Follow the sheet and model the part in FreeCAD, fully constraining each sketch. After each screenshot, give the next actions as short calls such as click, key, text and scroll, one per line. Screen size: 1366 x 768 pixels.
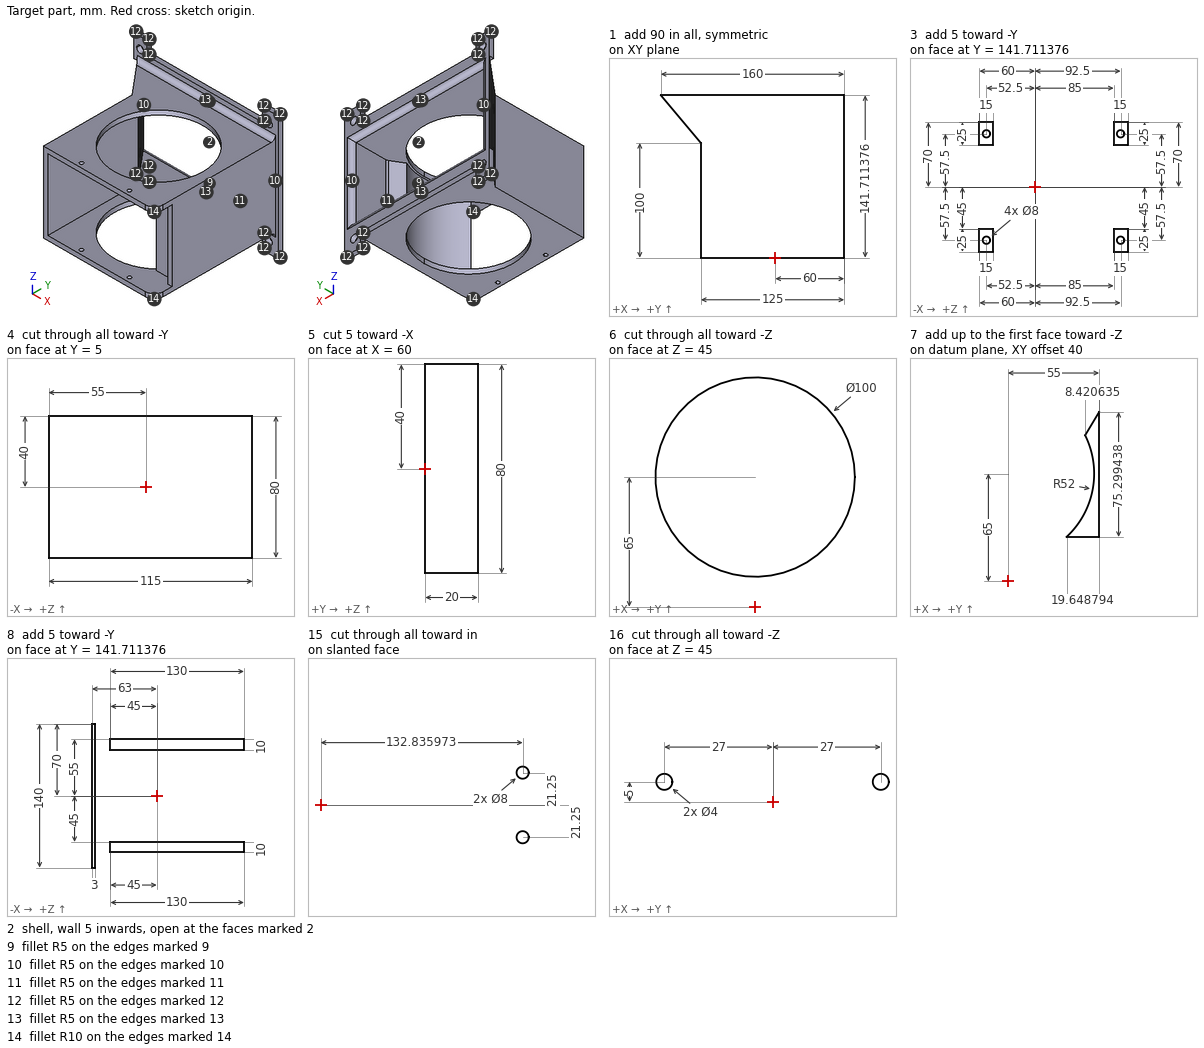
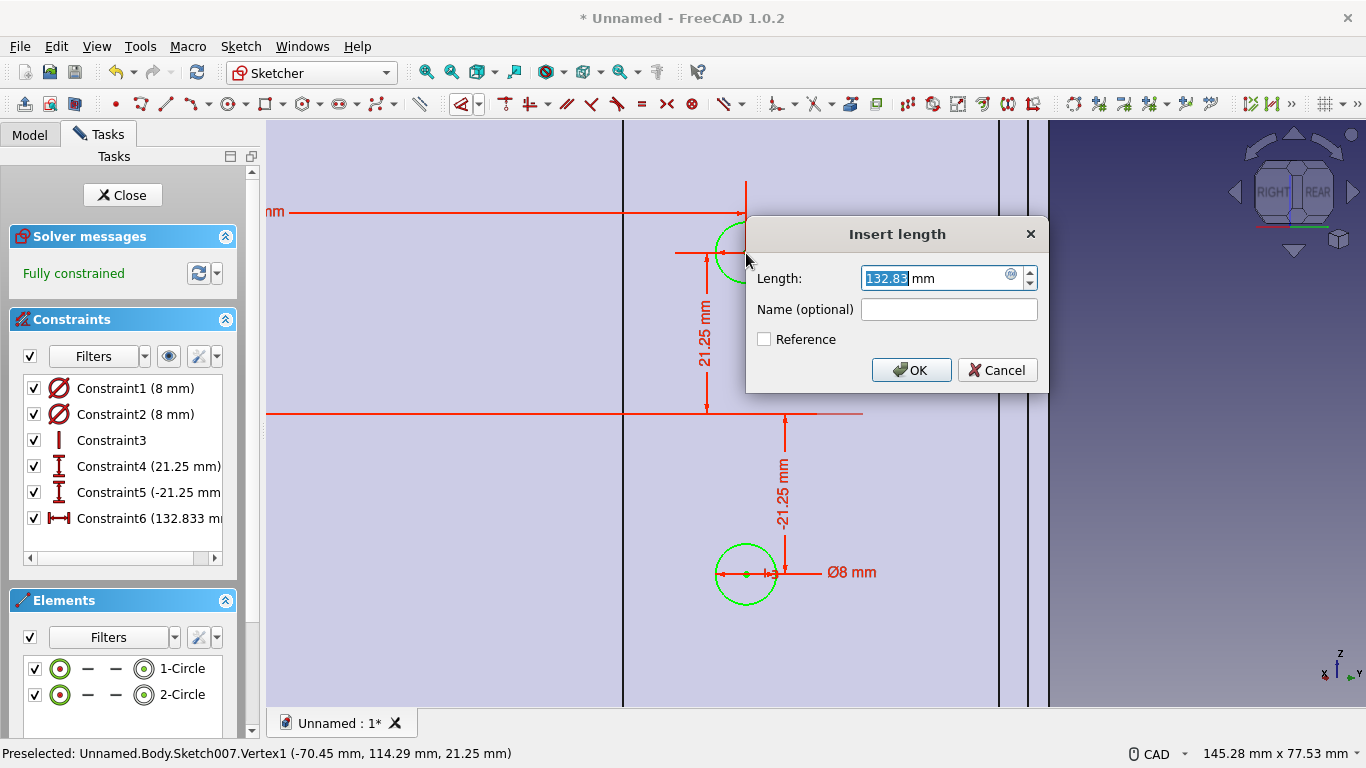
text(132.835973)
key(Return)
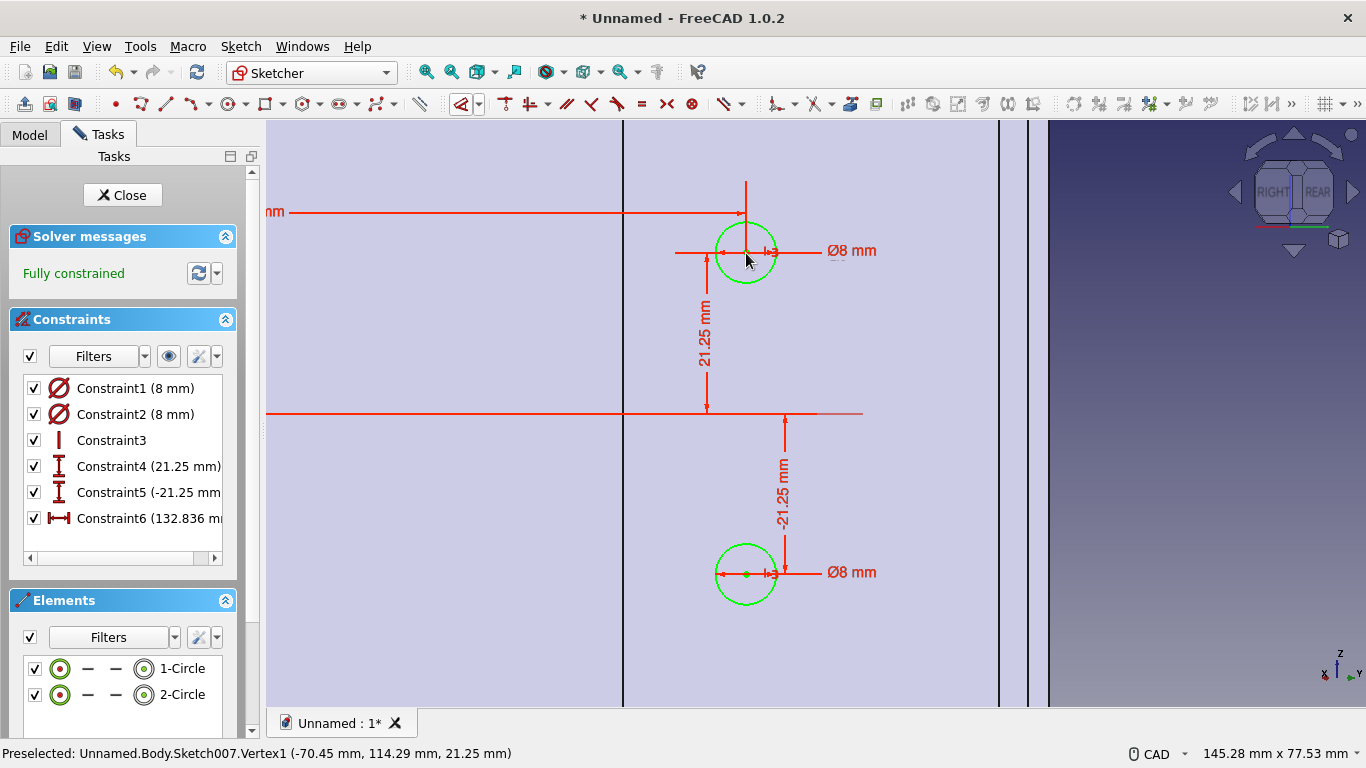
click(123, 195)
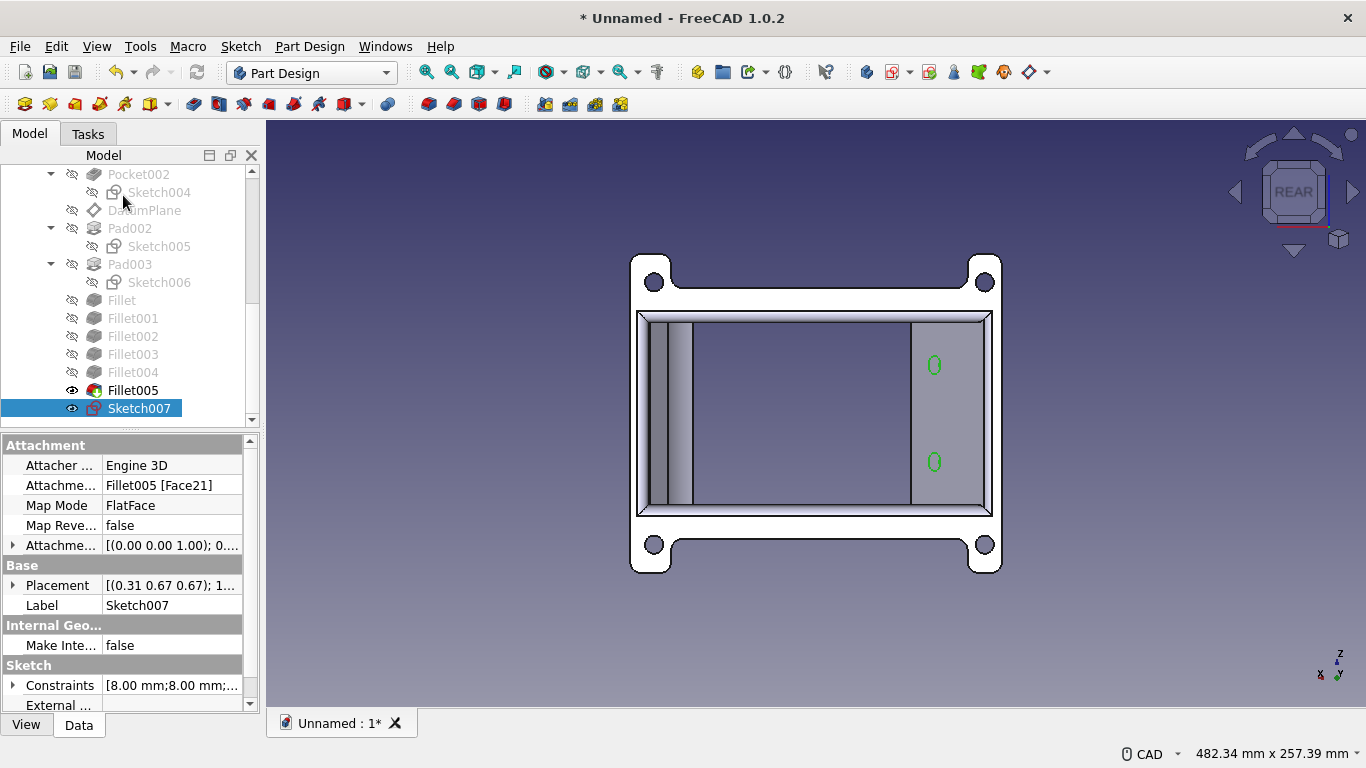
click(194, 104)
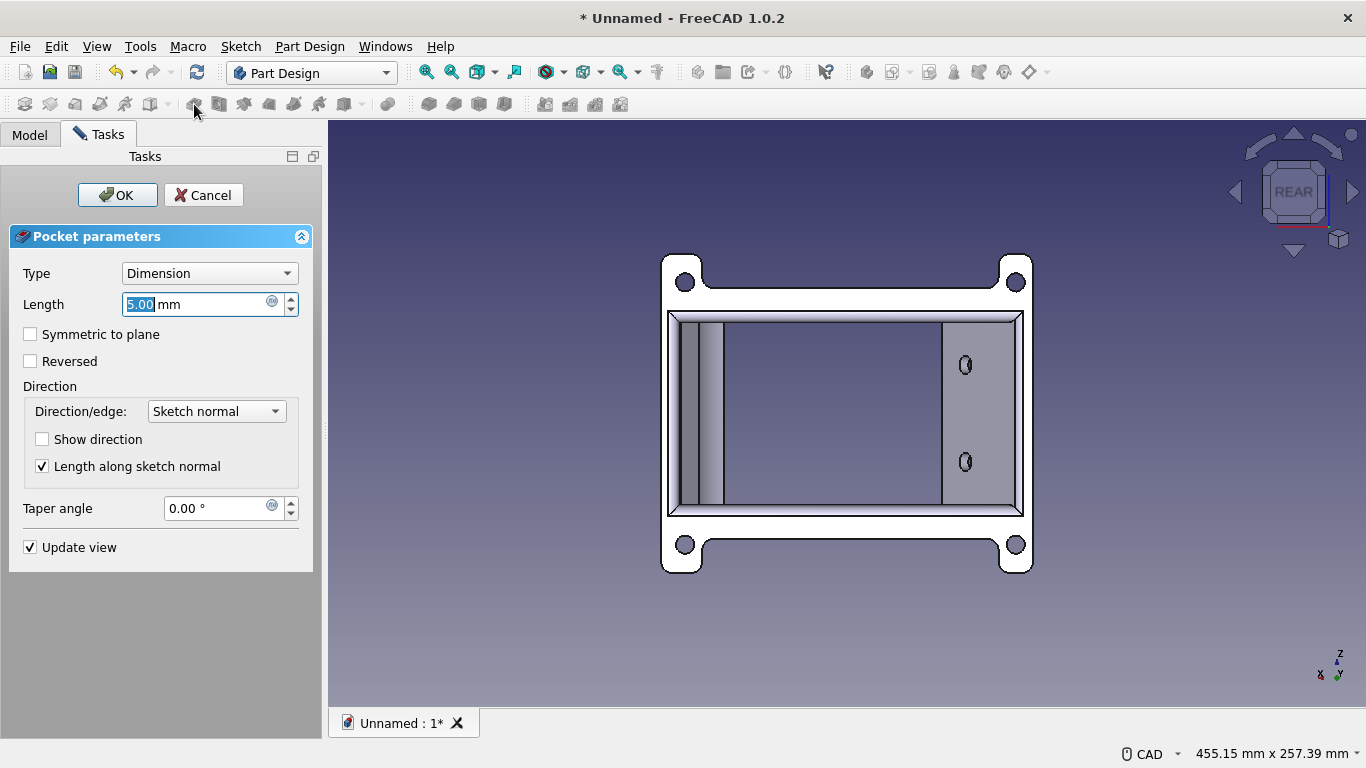
click(210, 274)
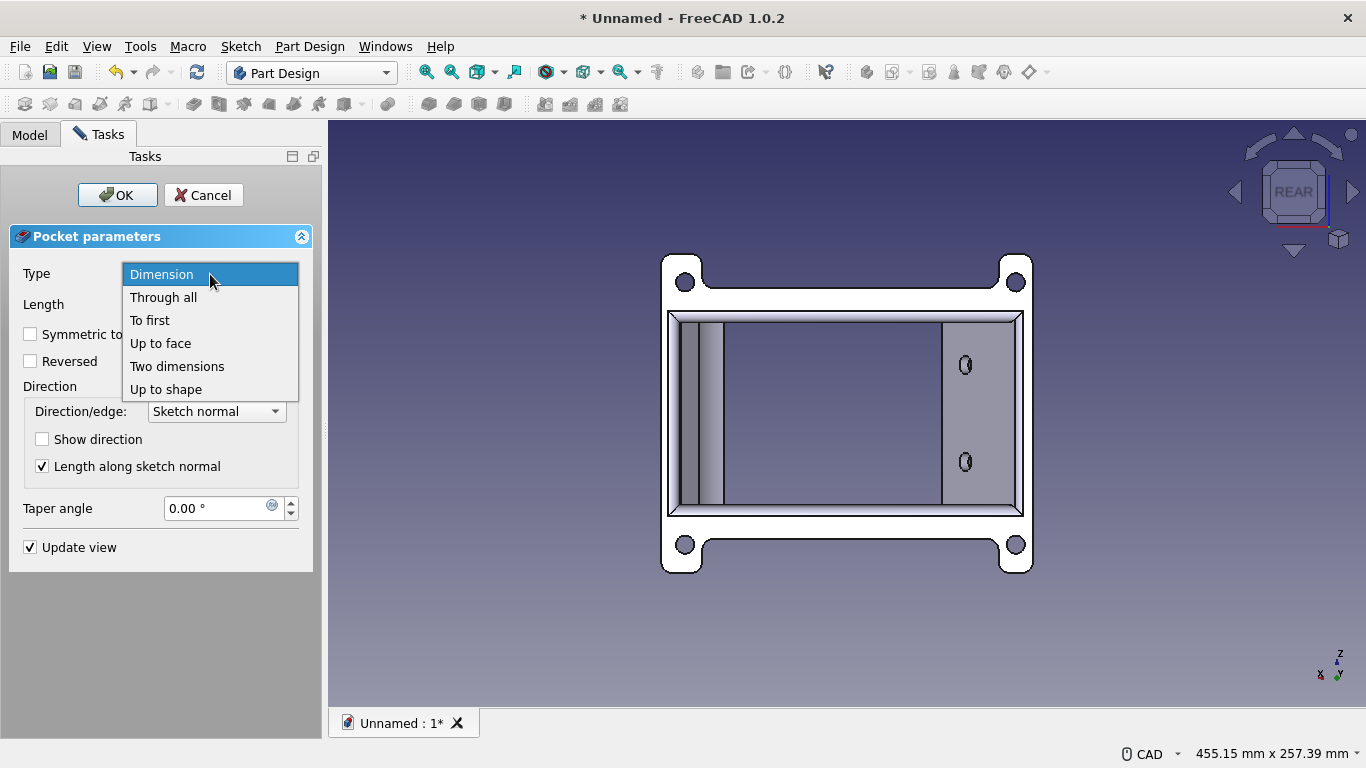
click(208, 298)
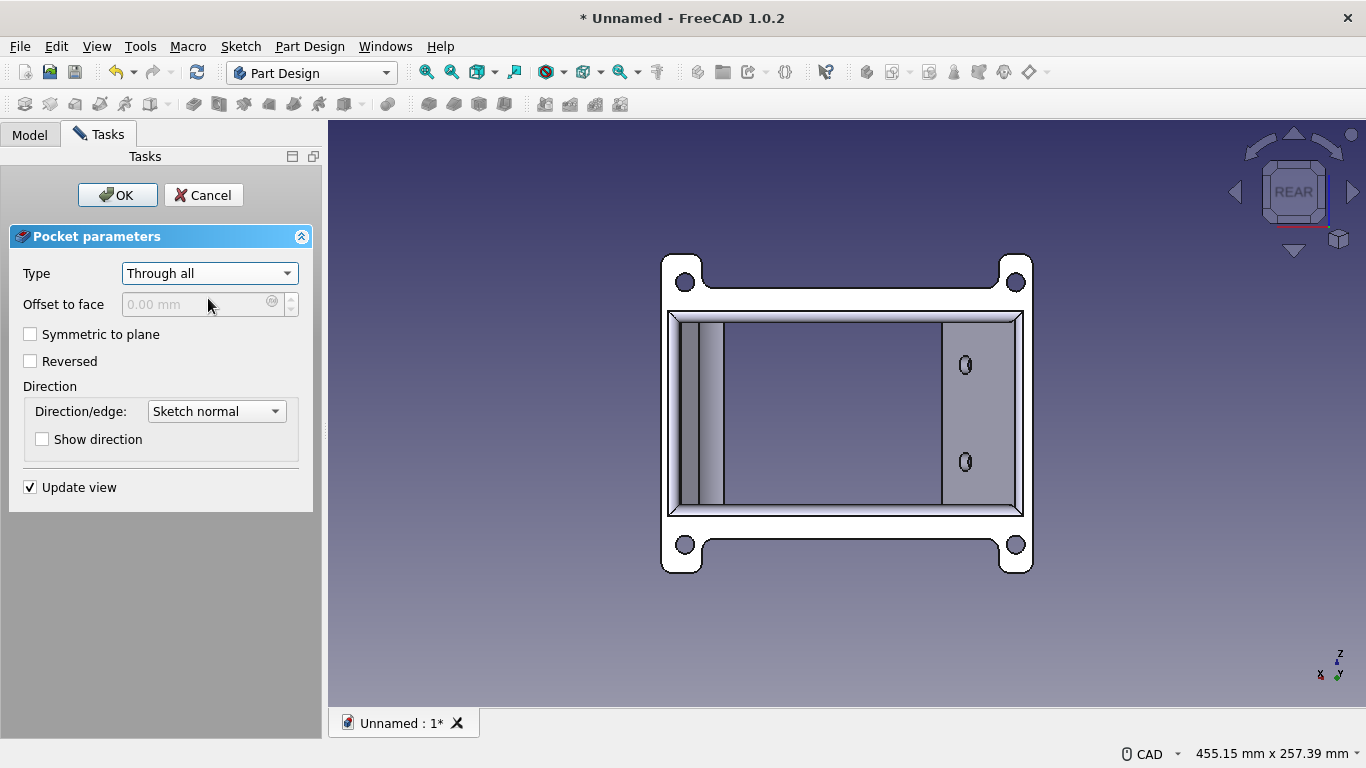
click(118, 195)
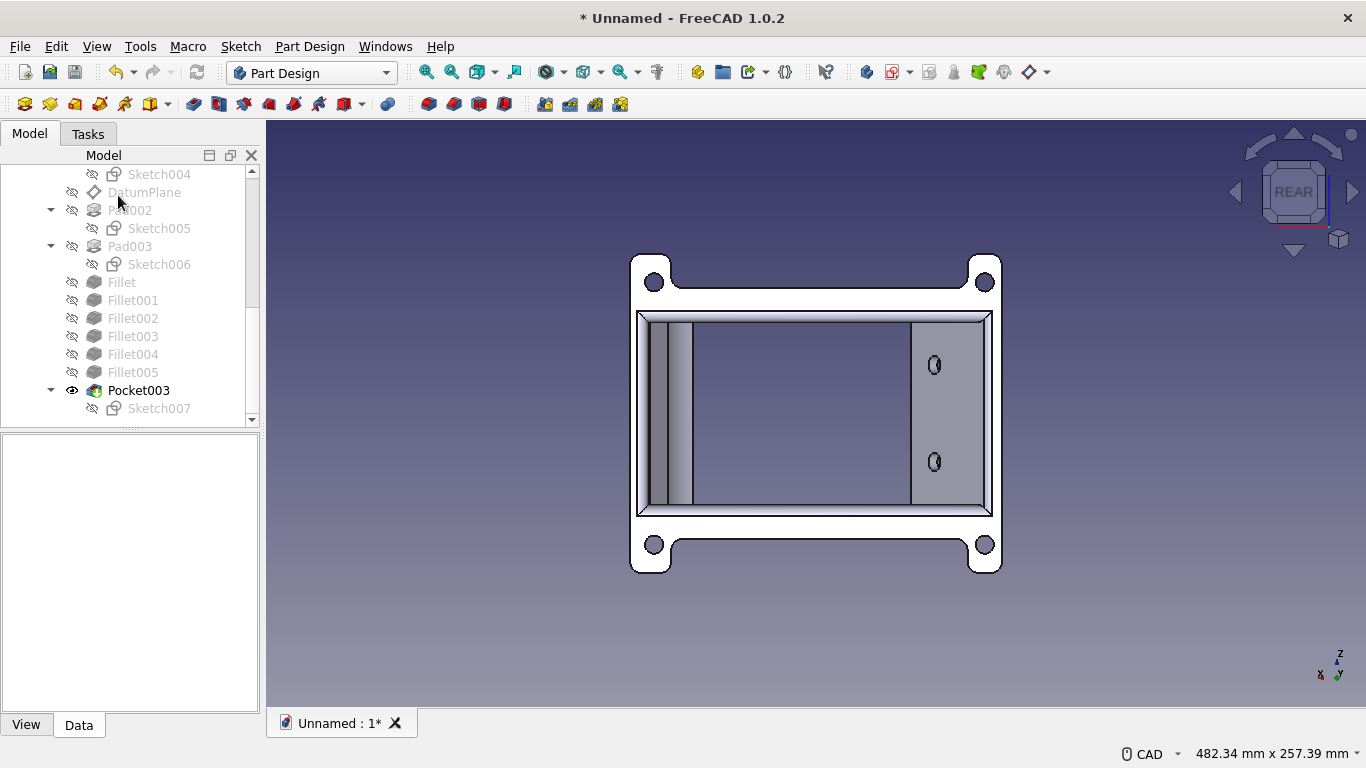
key(0)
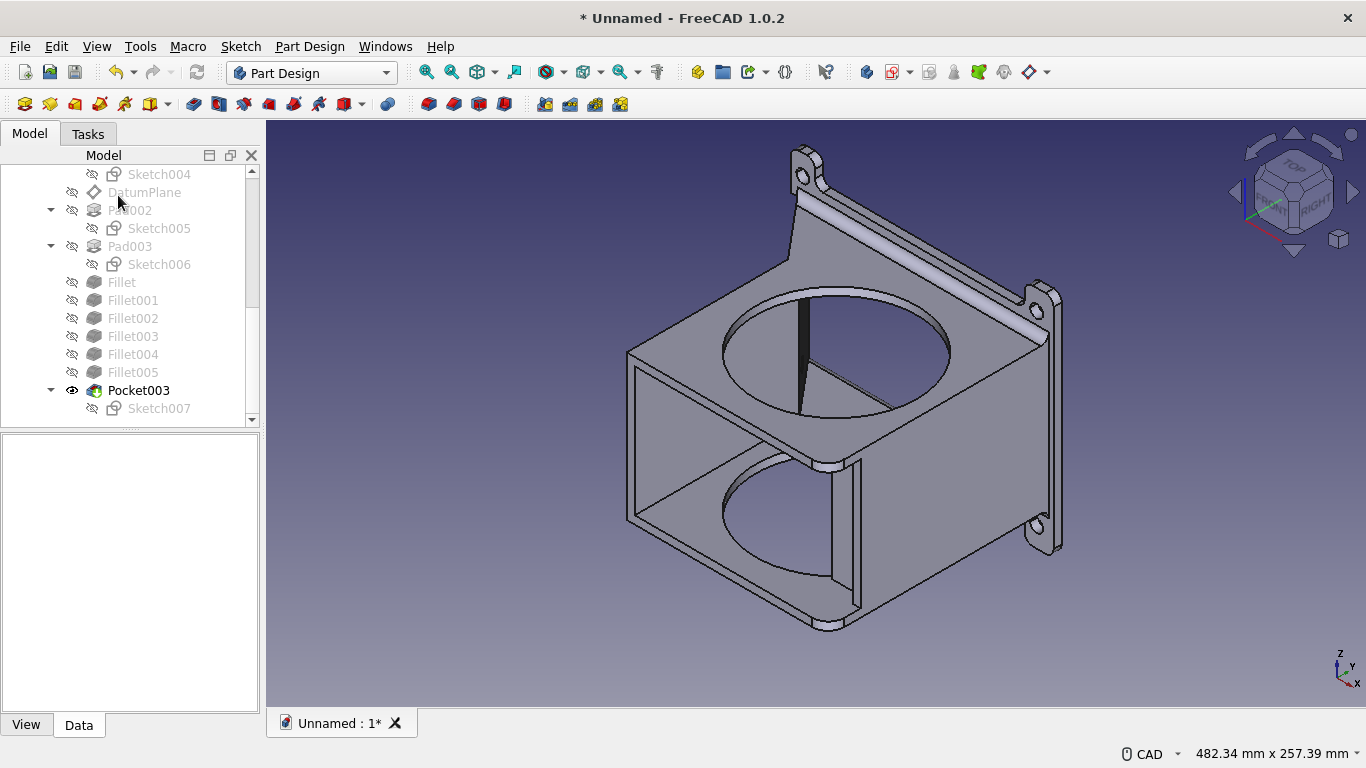
click(978, 361)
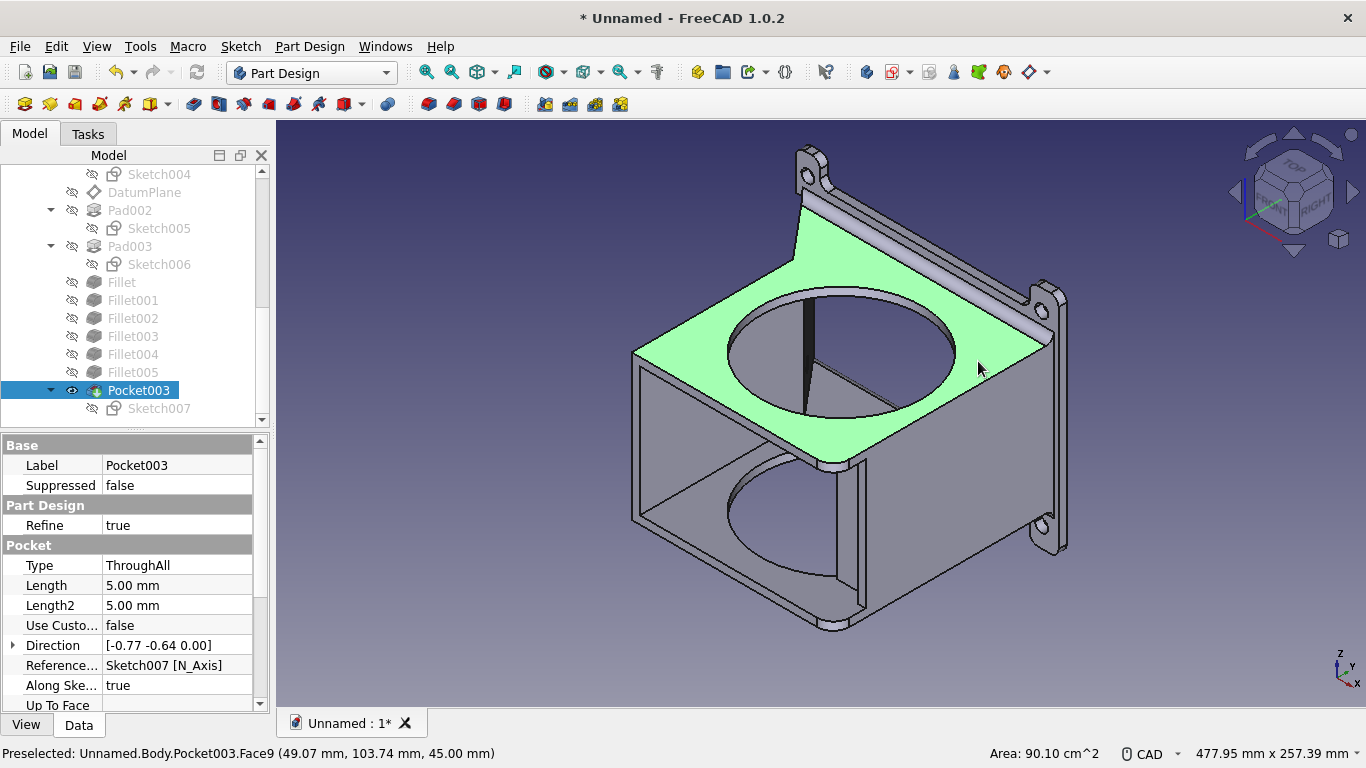
click(892, 72)